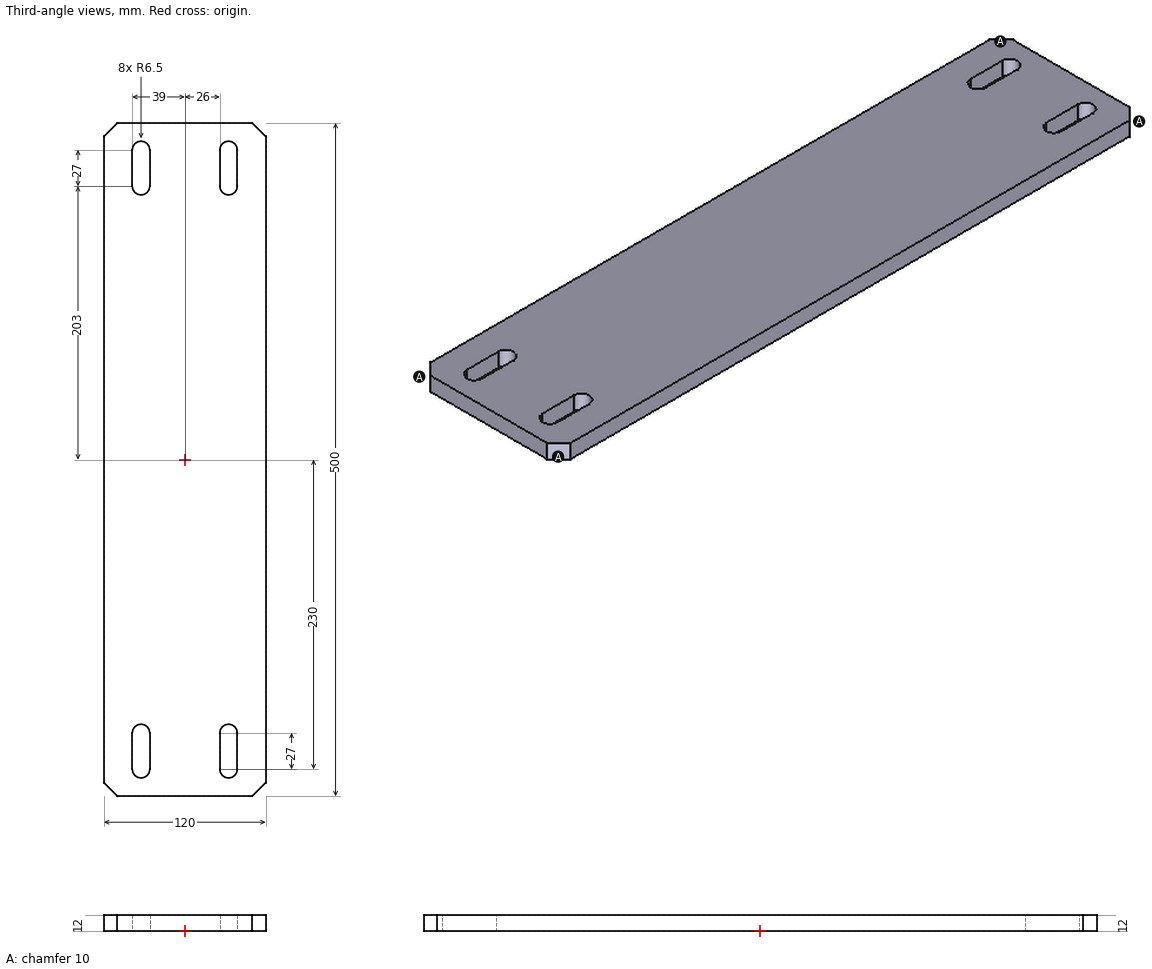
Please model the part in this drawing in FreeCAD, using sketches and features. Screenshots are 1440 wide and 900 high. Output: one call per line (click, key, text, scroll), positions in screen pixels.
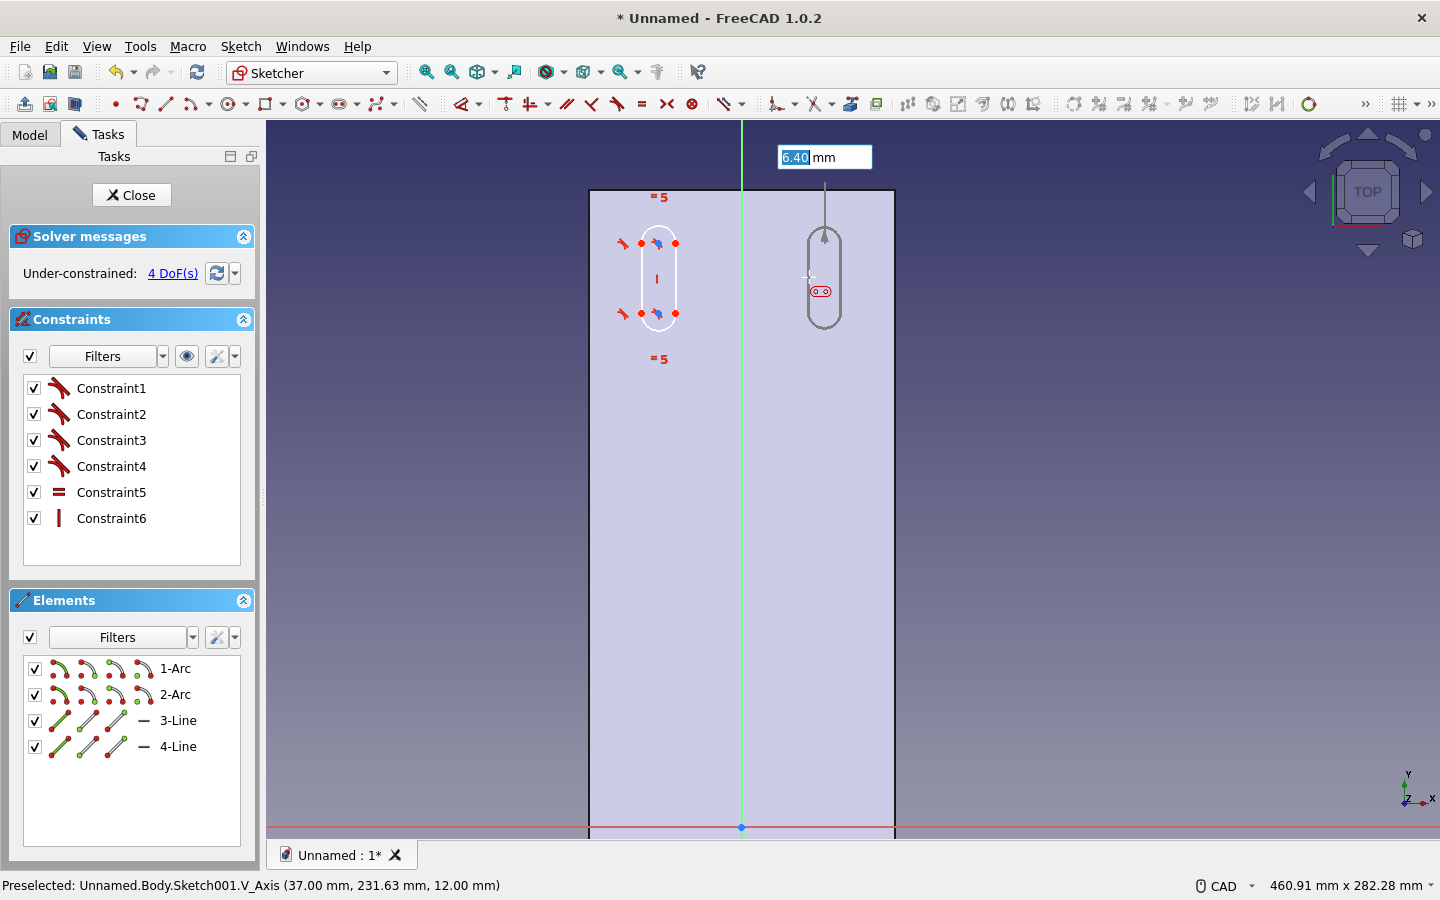
click(808, 276)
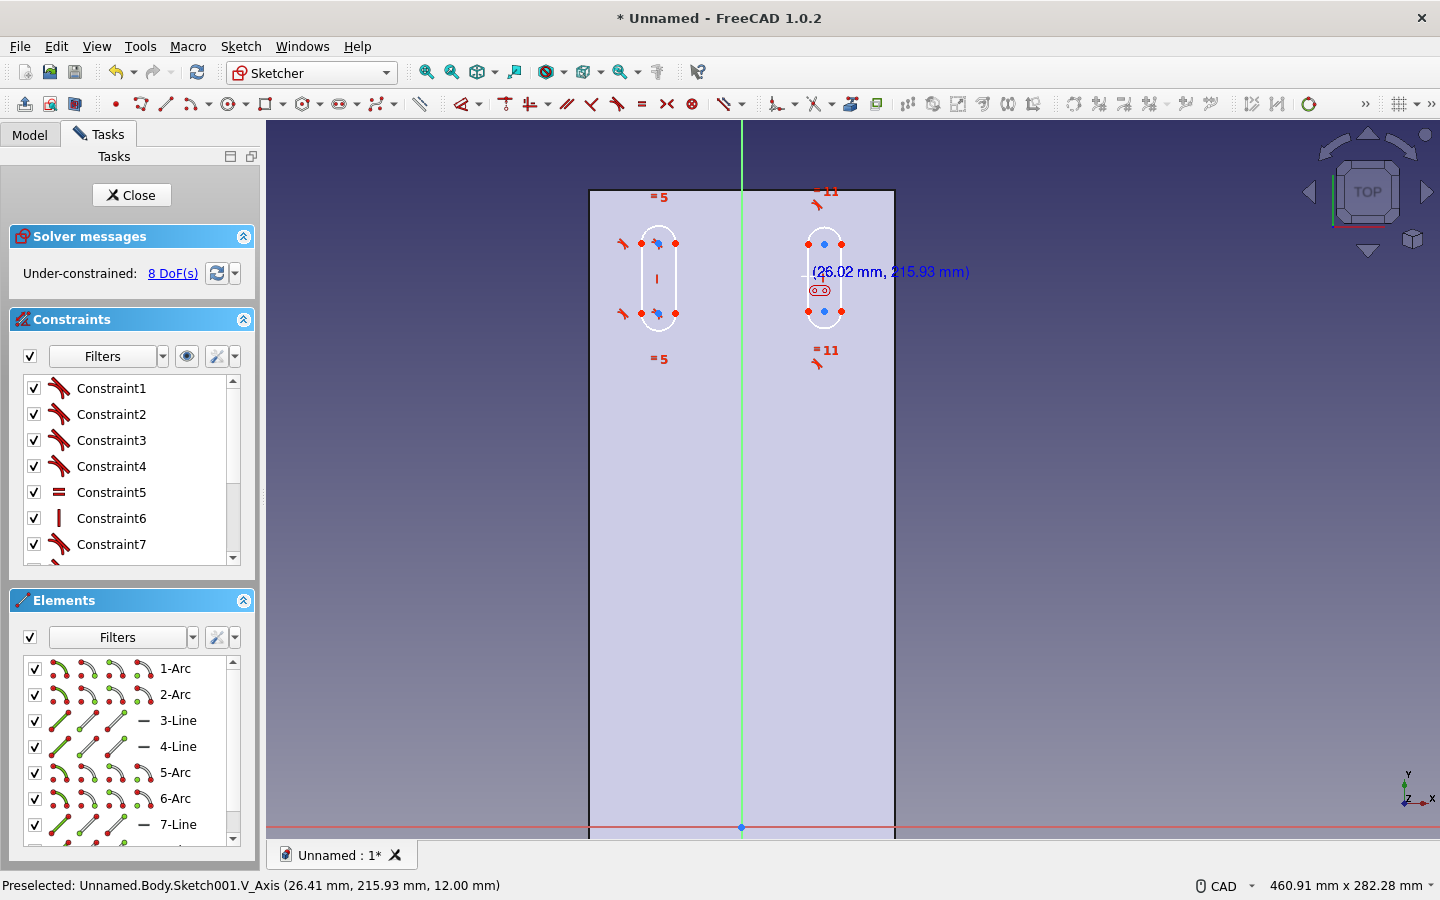
scroll(809, 277, down, 5)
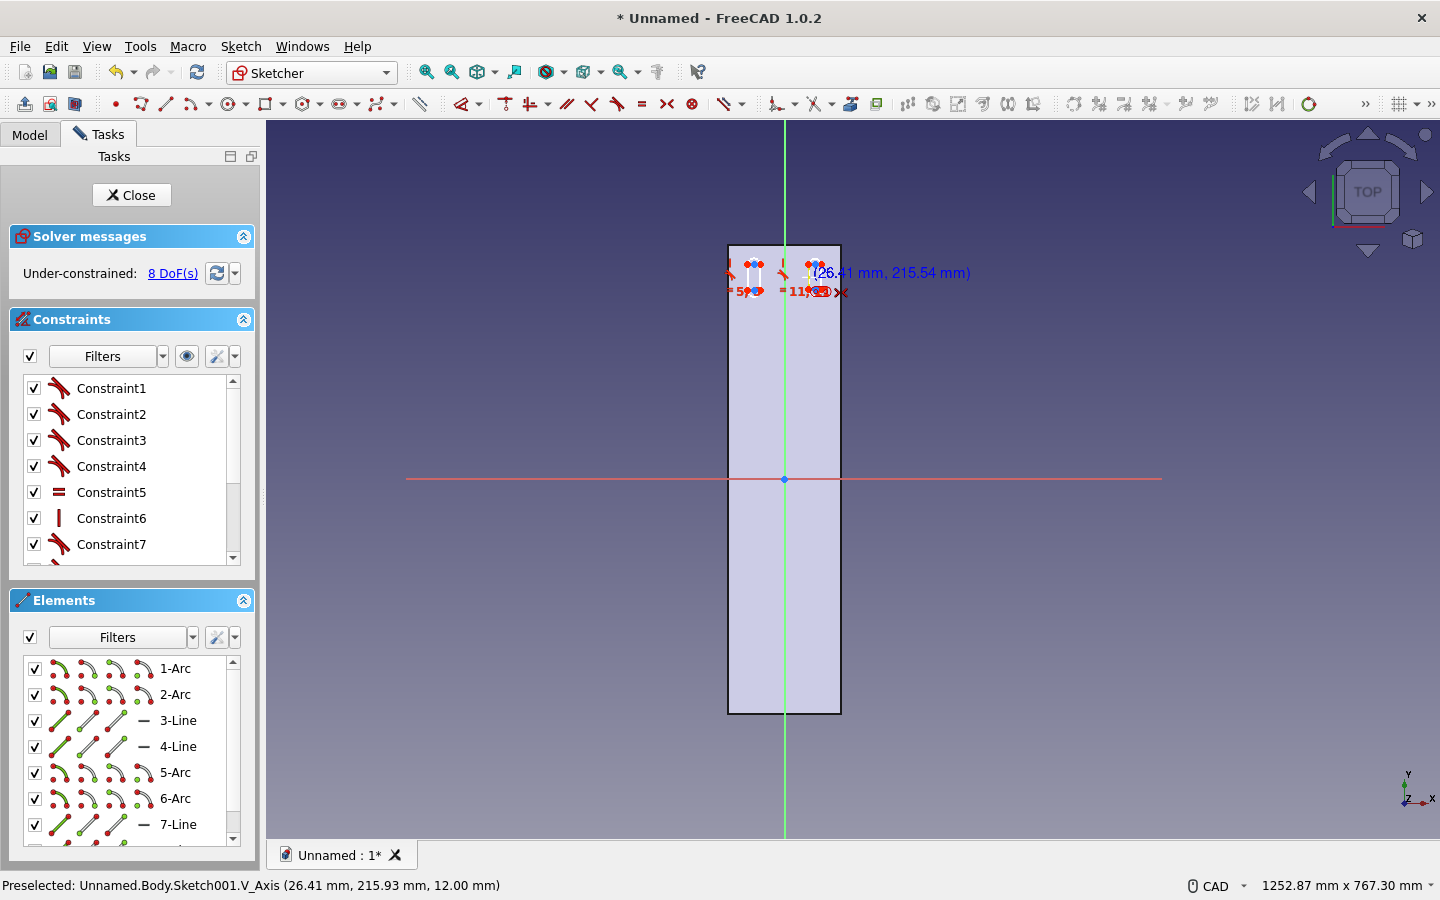
scroll(815, 695, up, 7)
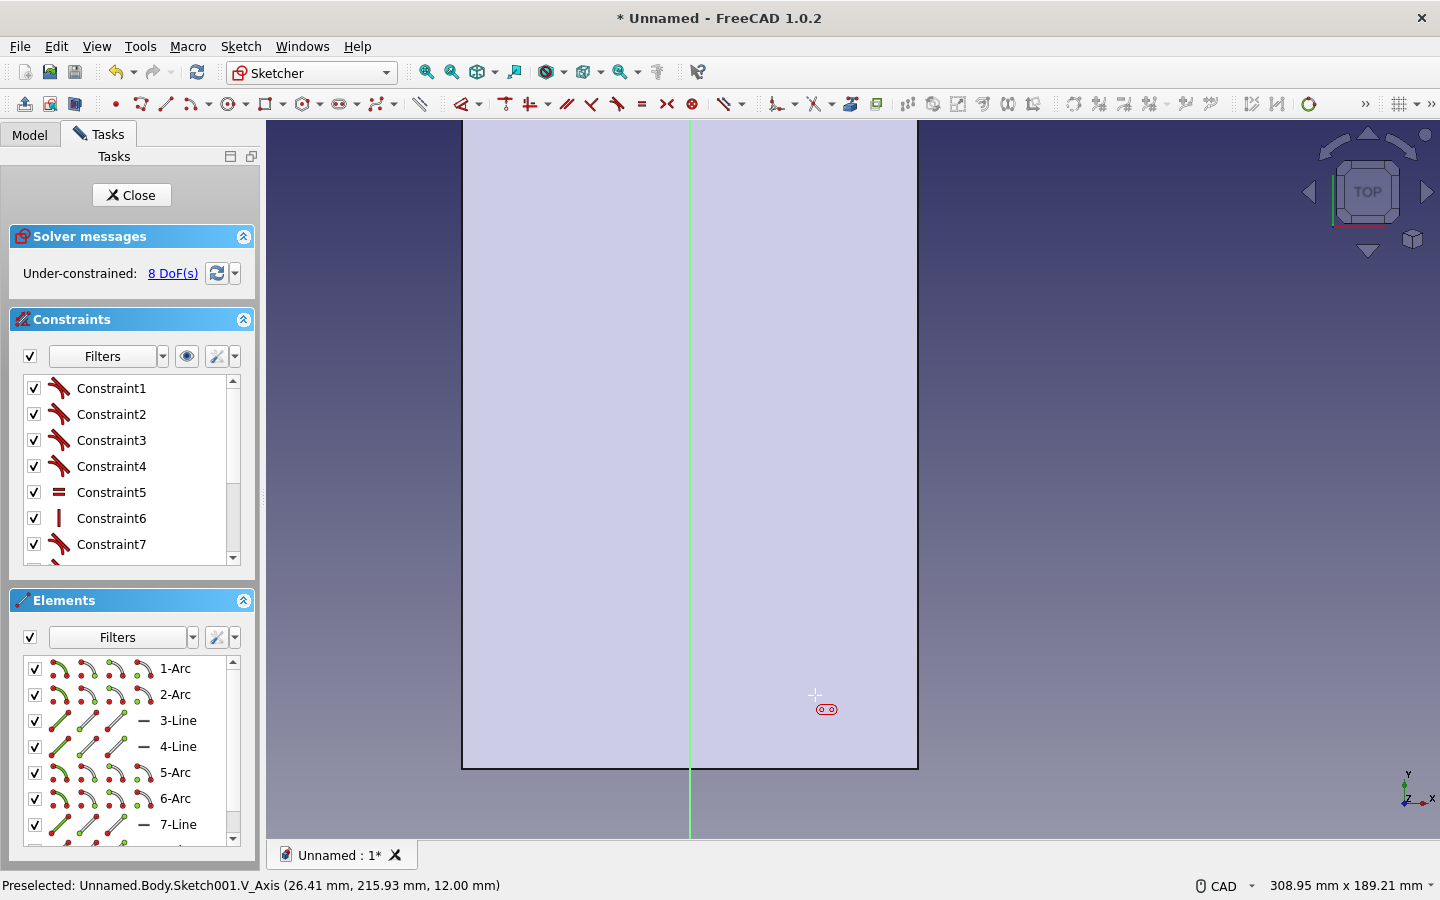
scroll(815, 696, down, 7)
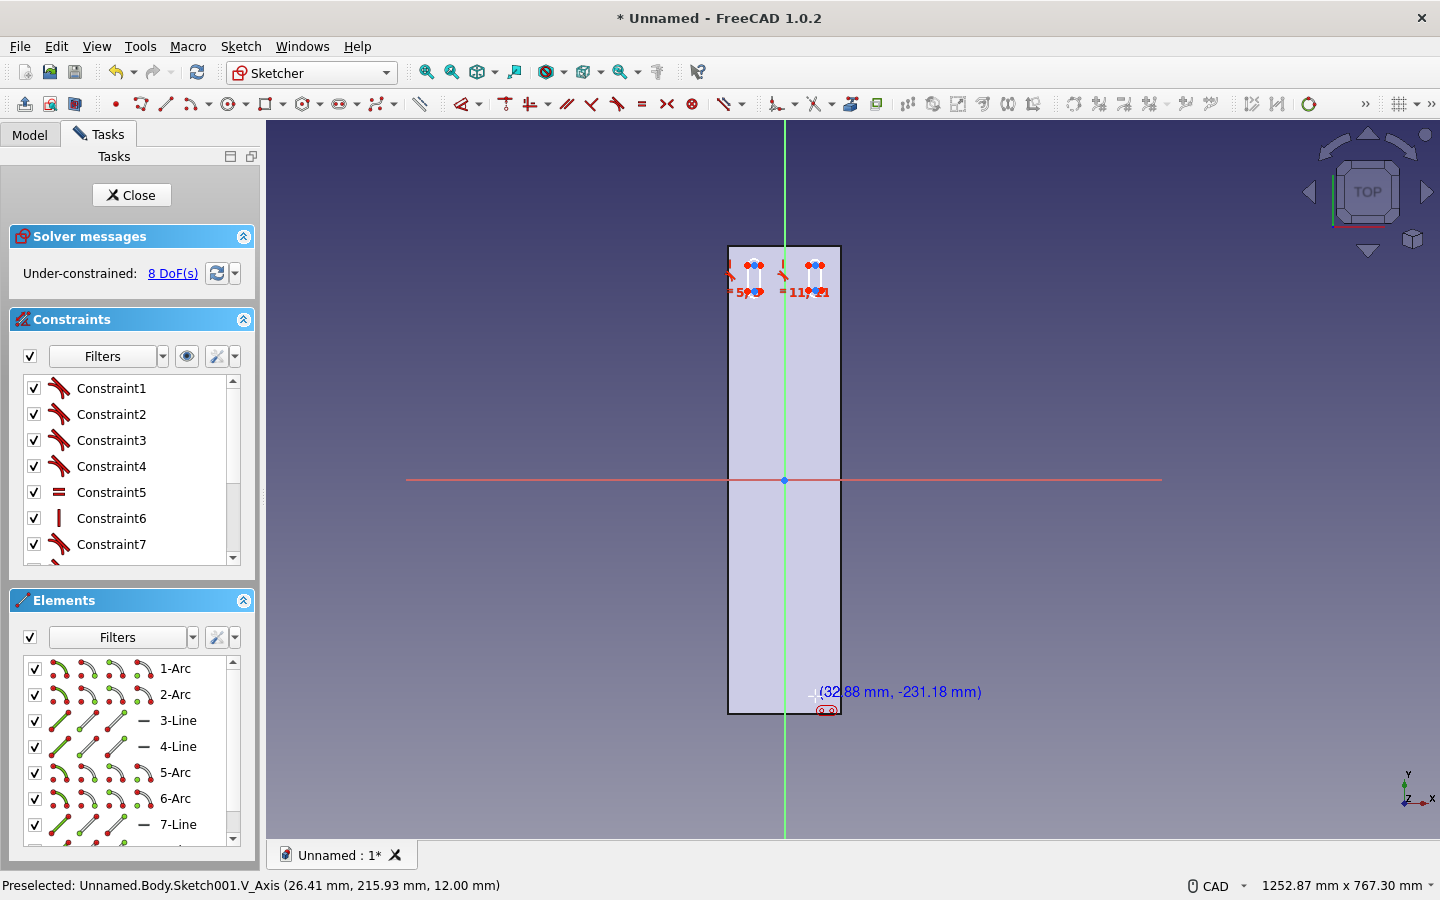
click(815, 696)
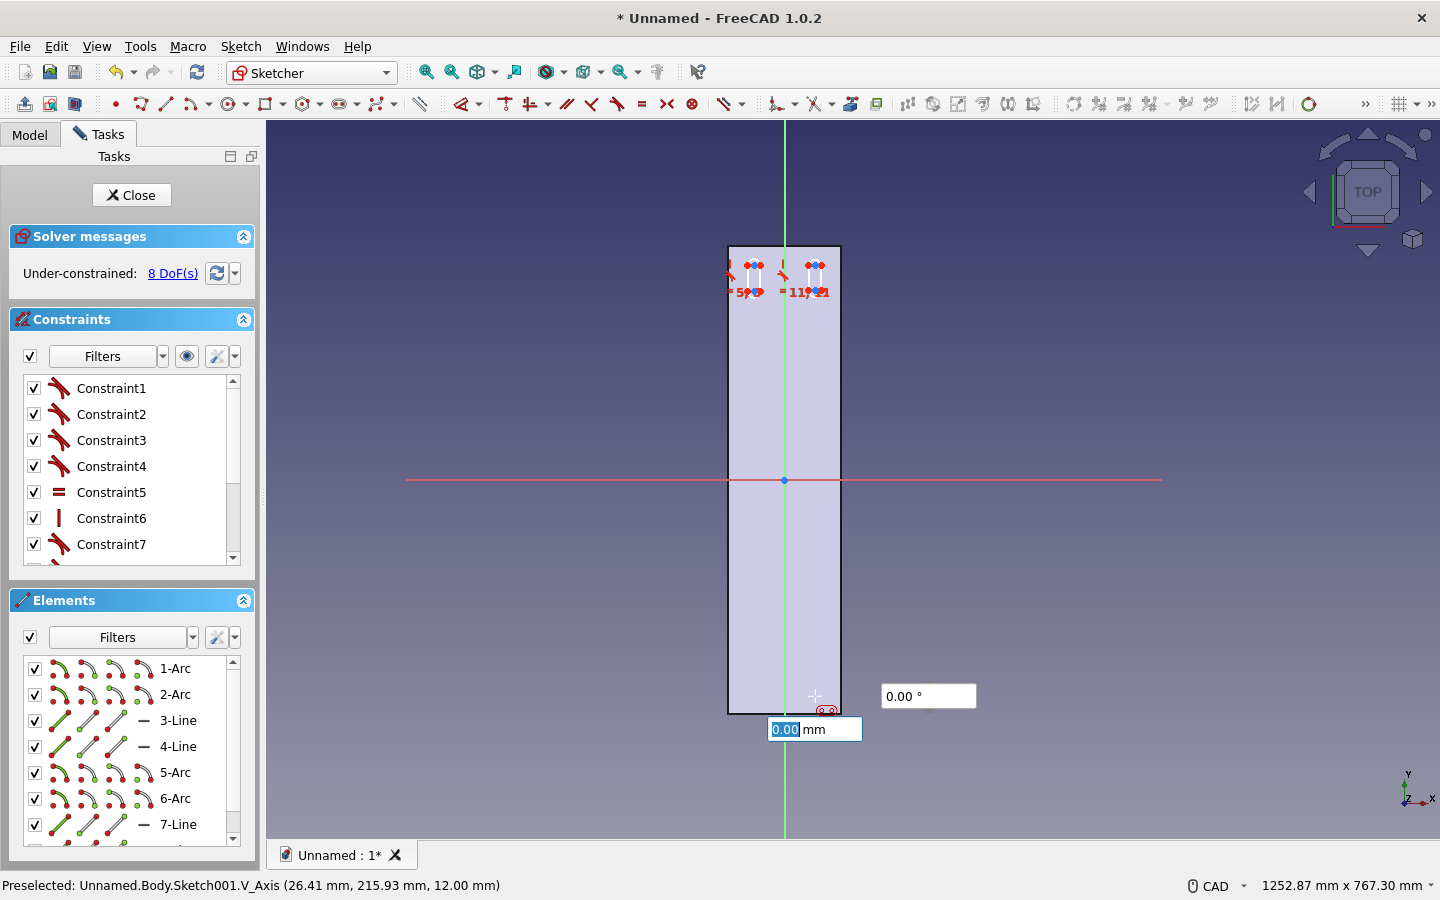
click(815, 670)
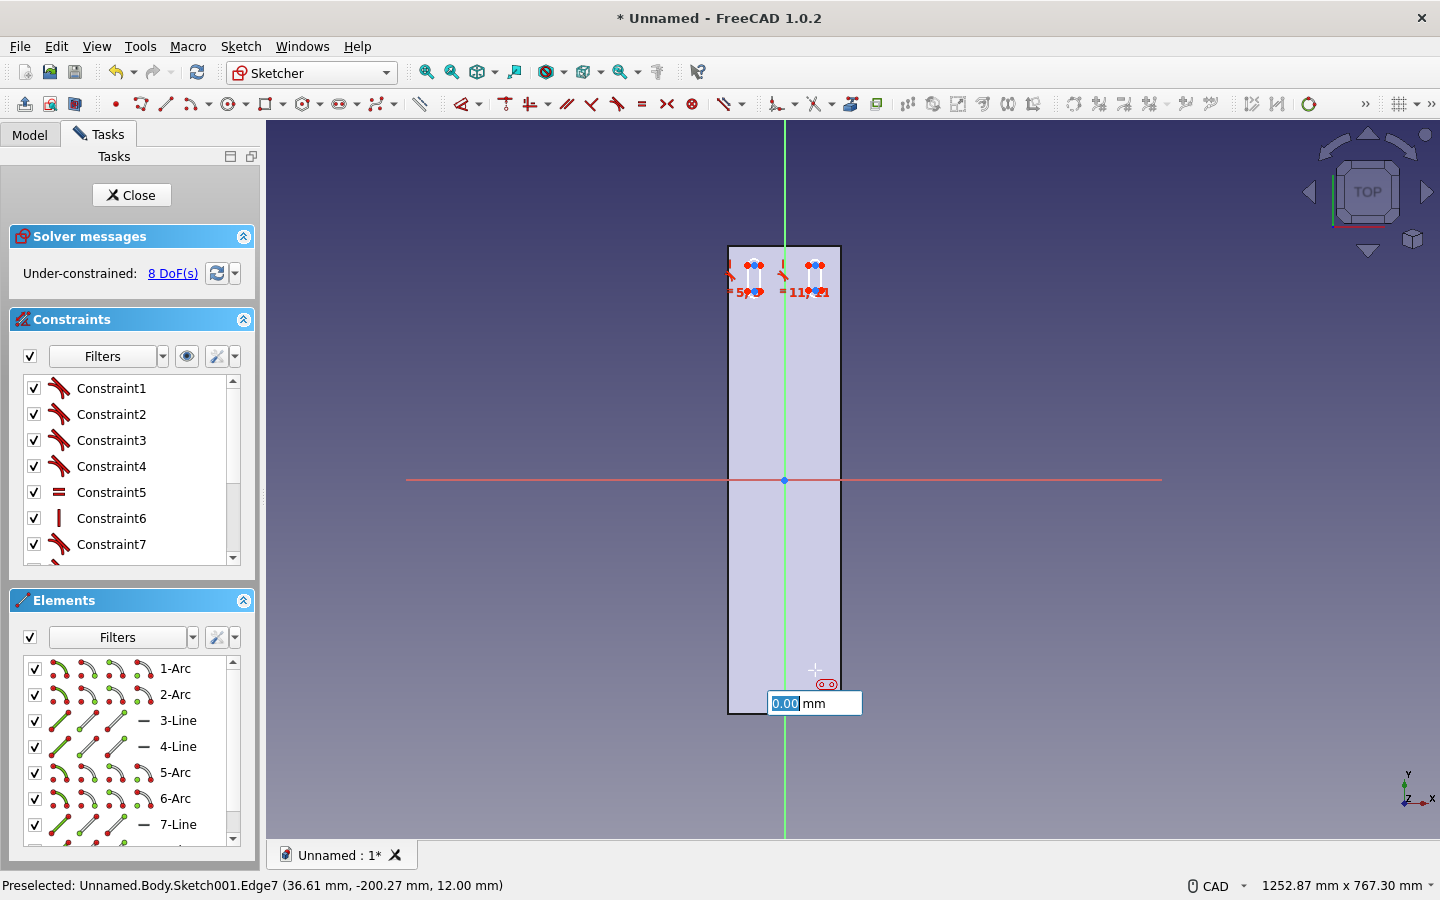
scroll(809, 683, up, 5)